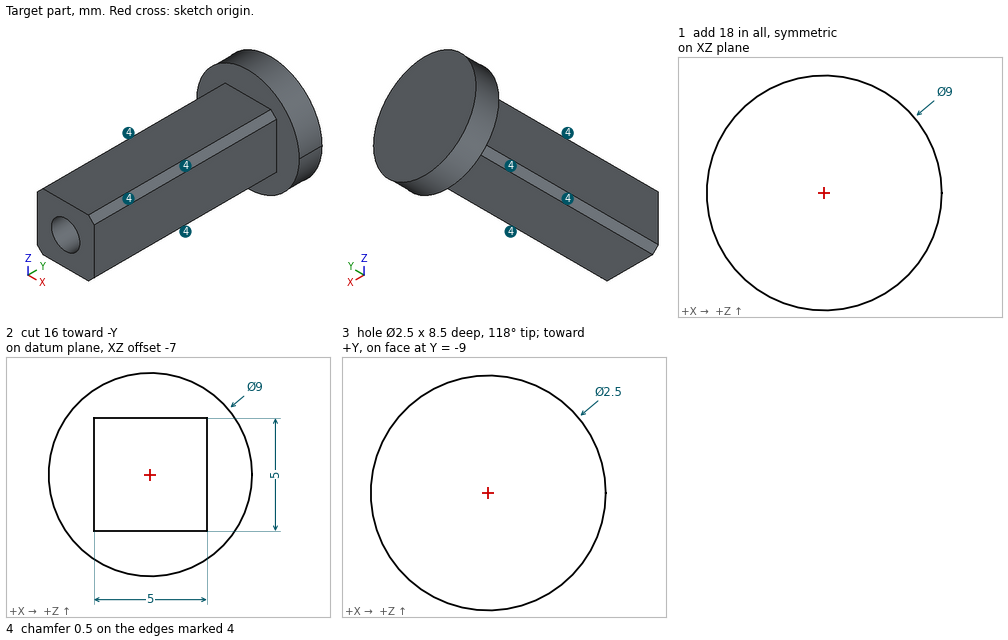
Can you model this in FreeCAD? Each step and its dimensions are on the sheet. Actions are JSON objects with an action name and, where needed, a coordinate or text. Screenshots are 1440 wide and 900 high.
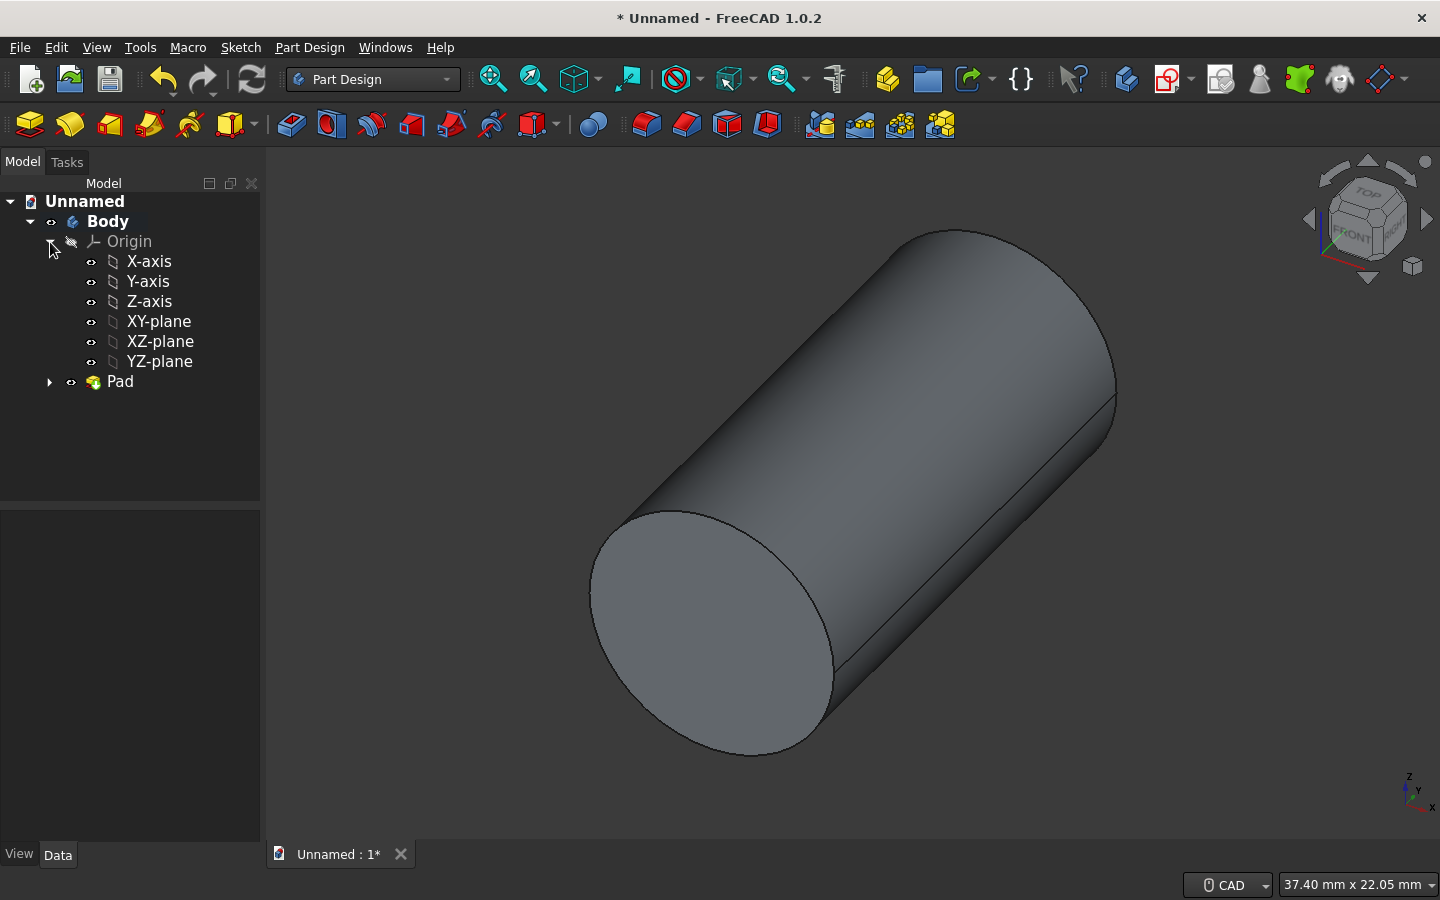
{"action": "left_click", "coordinate": [136, 342]}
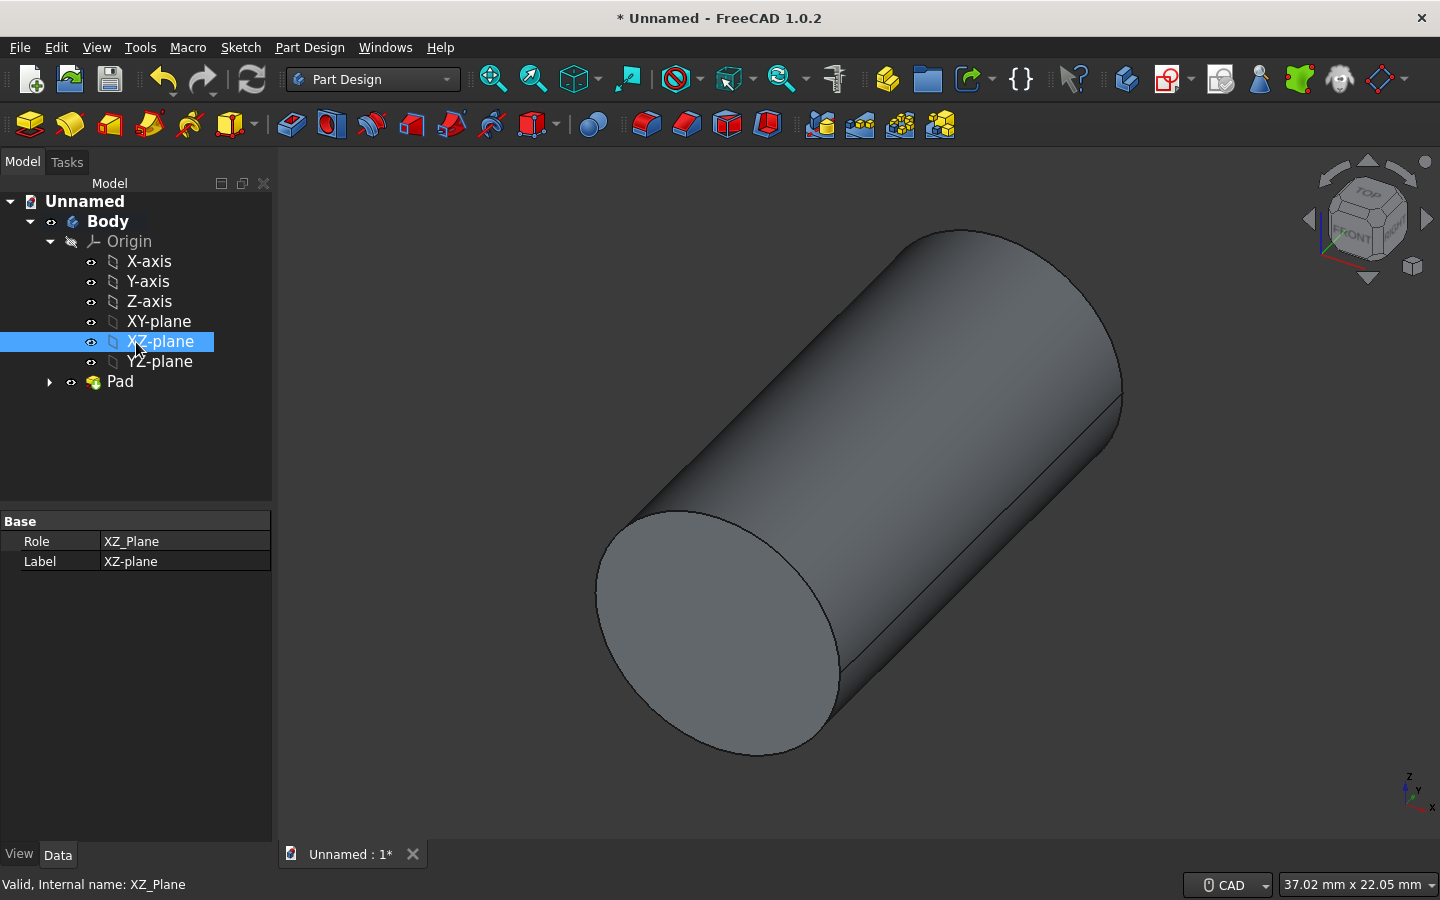
{"action": "left_click", "coordinate": [1380, 80]}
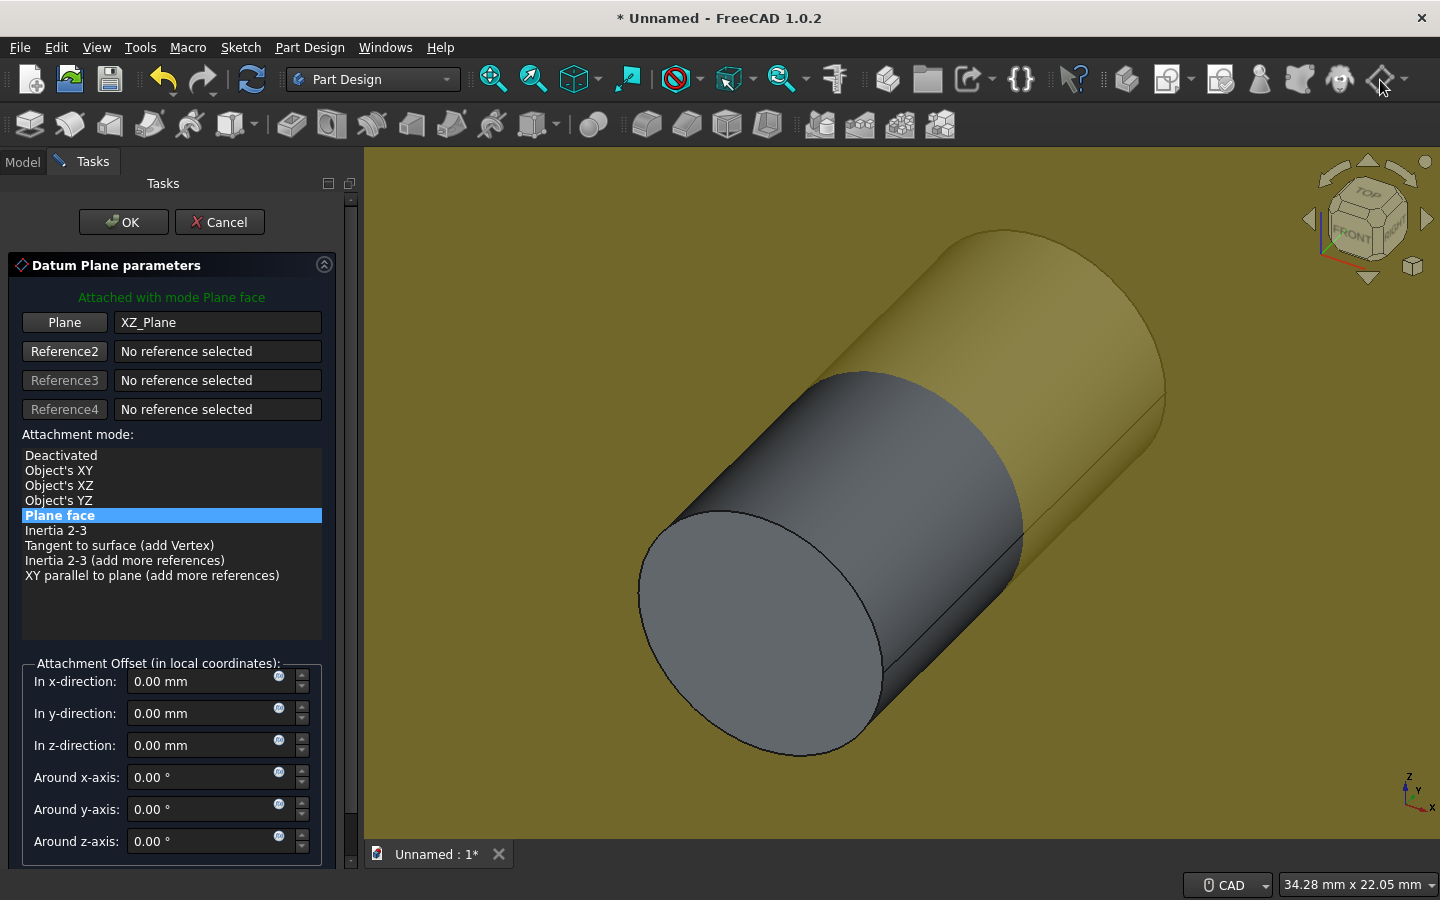
{"action": "triple_click", "coordinate": [210, 745]}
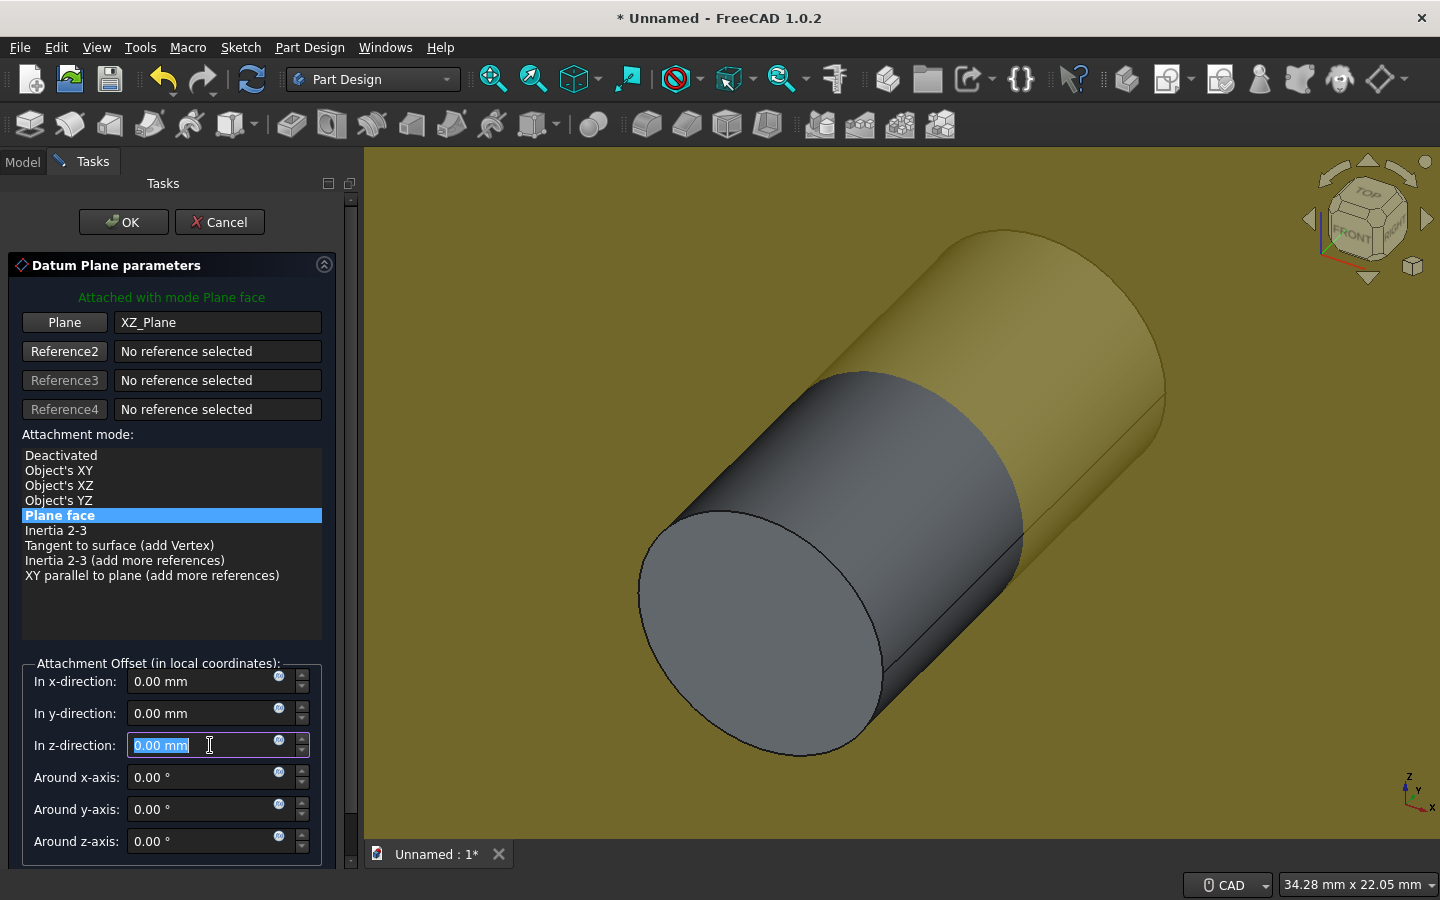
{"action": "type", "text": "-7"}
{"action": "key", "text": "Tab"}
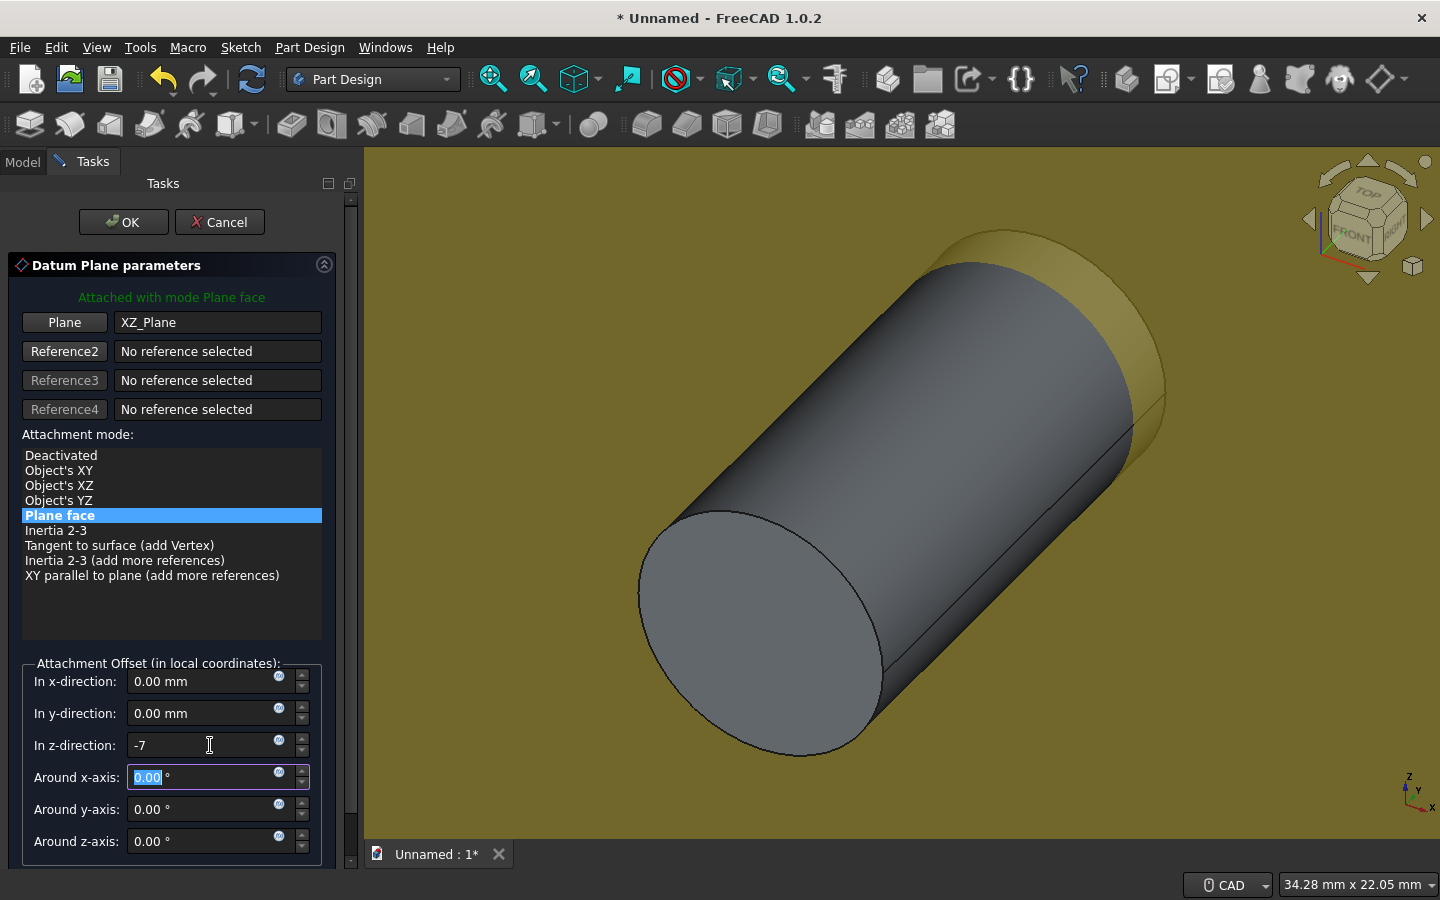
{"action": "left_click", "coordinate": [124, 222]}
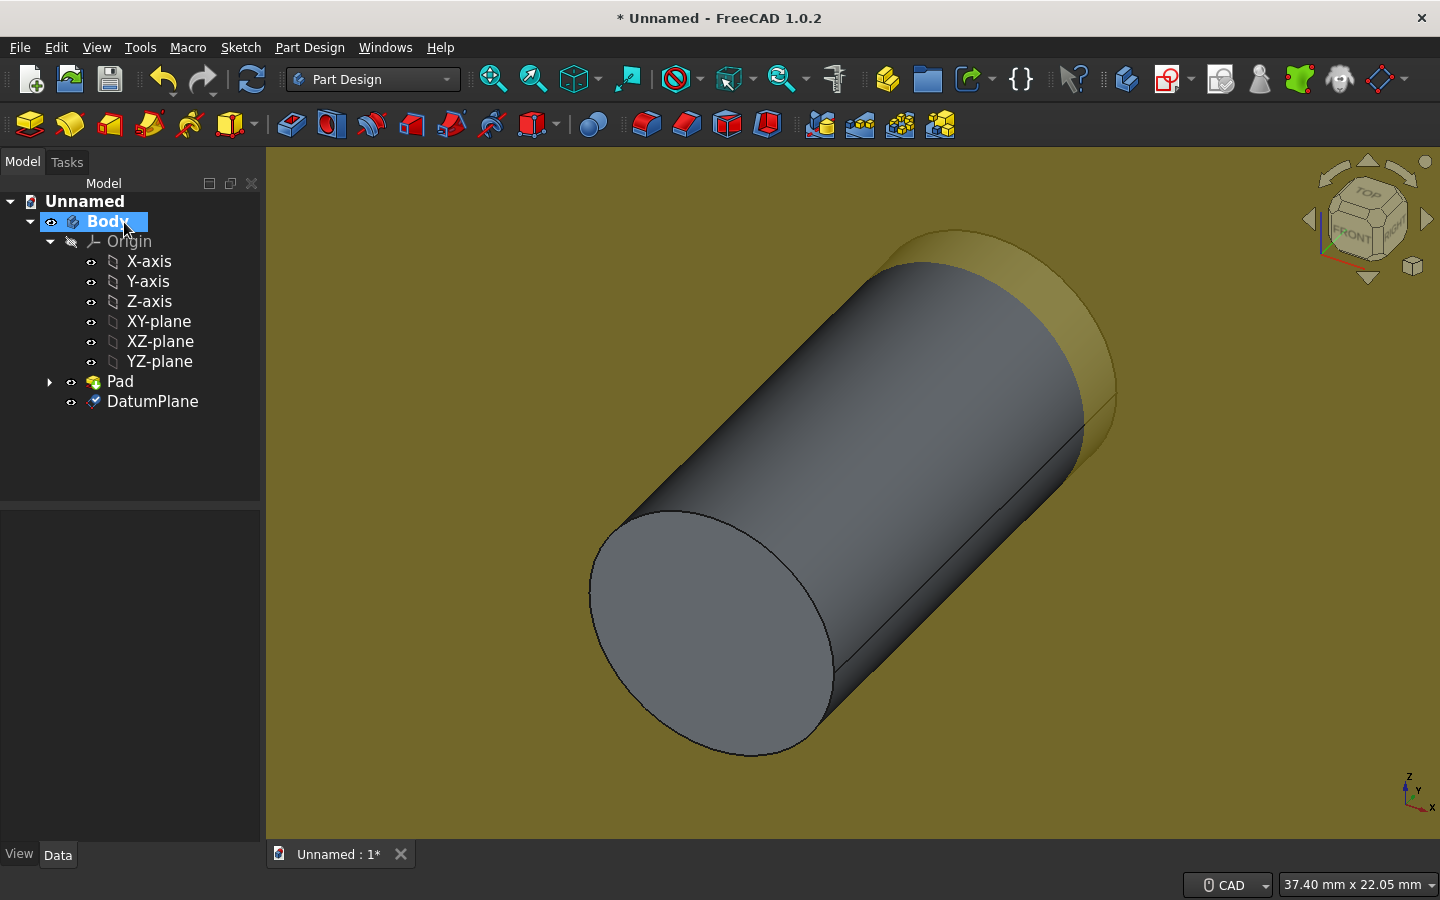
{"action": "left_click", "coordinate": [116, 402]}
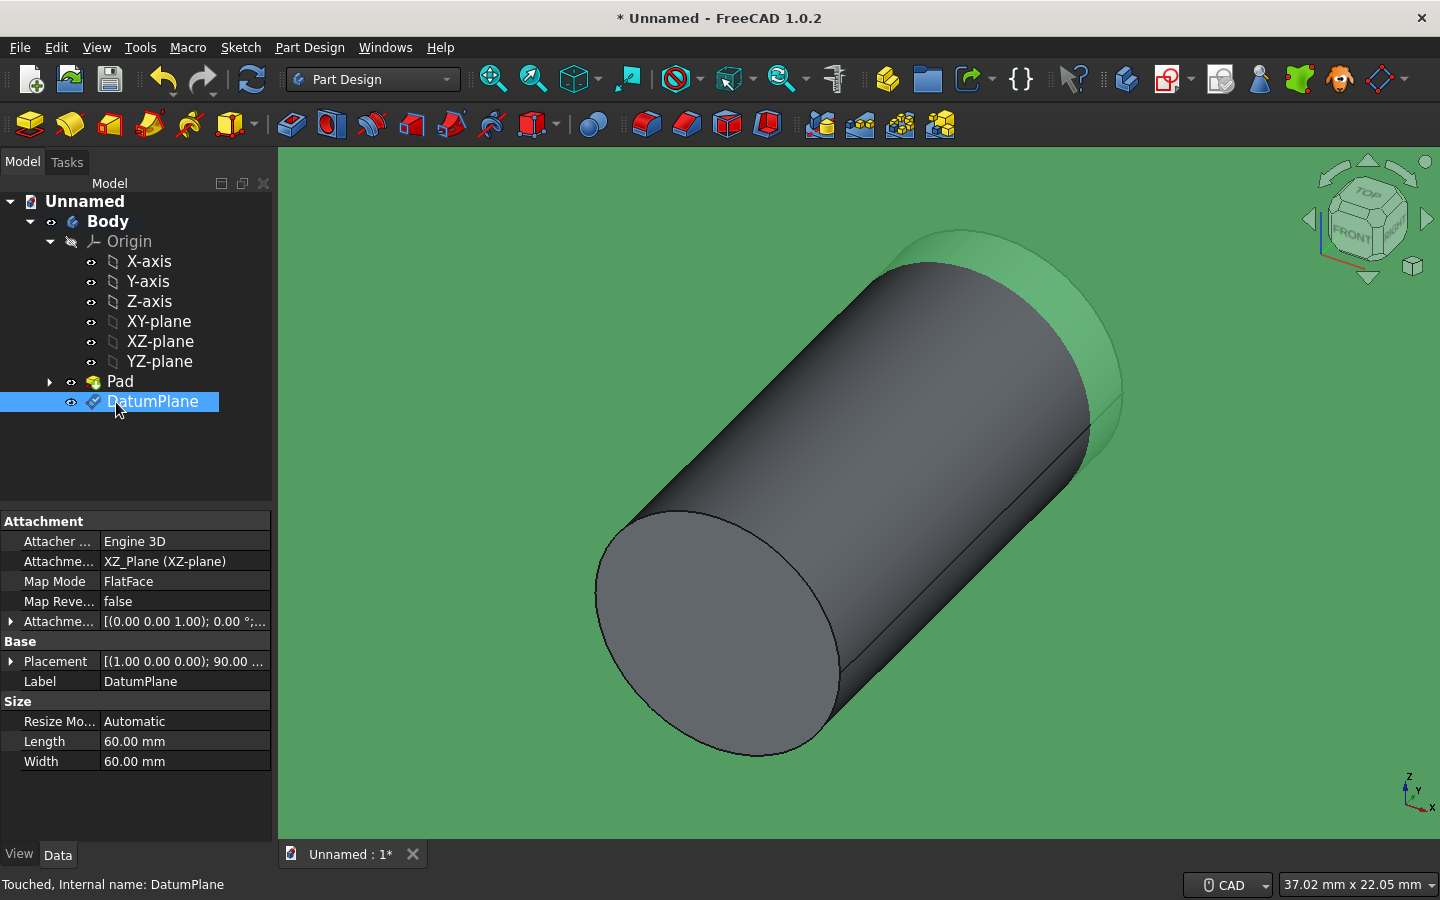
{"action": "left_click", "coordinate": [1168, 80]}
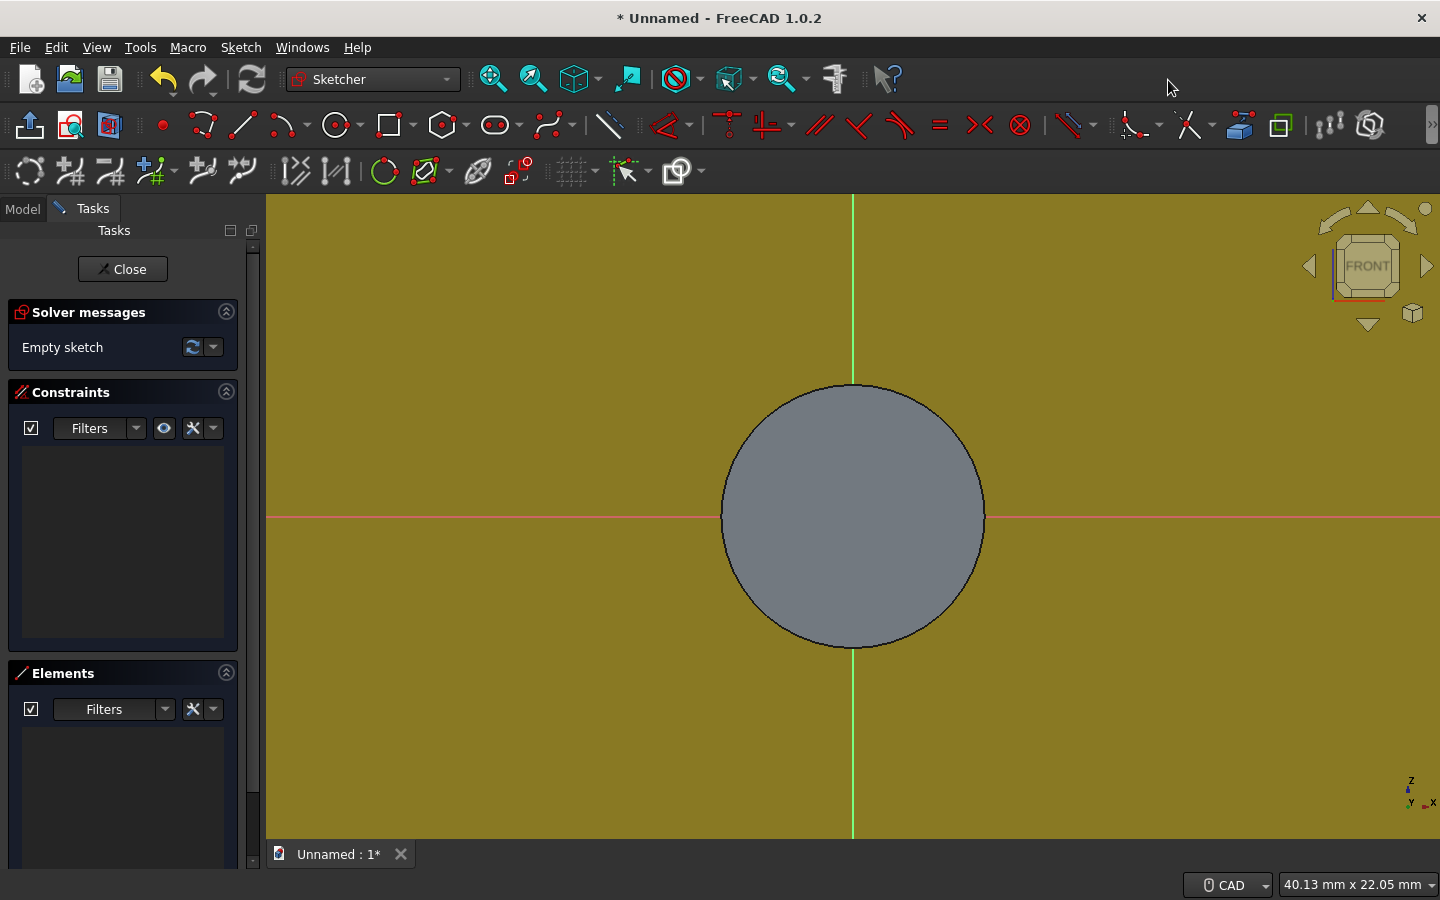
{"action": "left_click", "coordinate": [110, 126]}